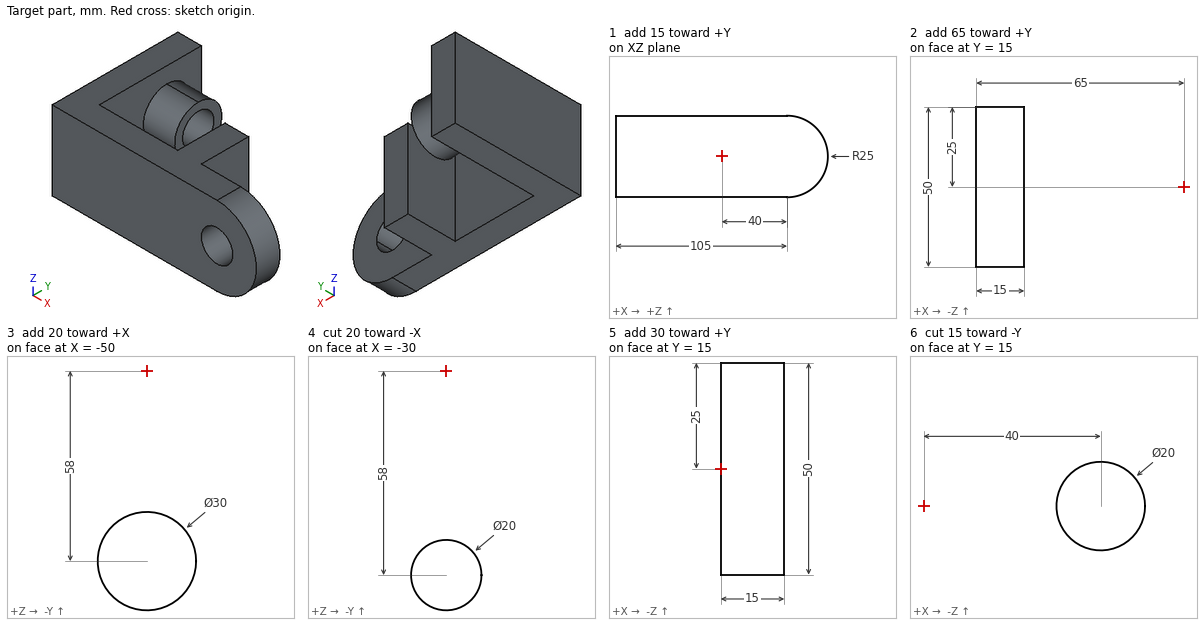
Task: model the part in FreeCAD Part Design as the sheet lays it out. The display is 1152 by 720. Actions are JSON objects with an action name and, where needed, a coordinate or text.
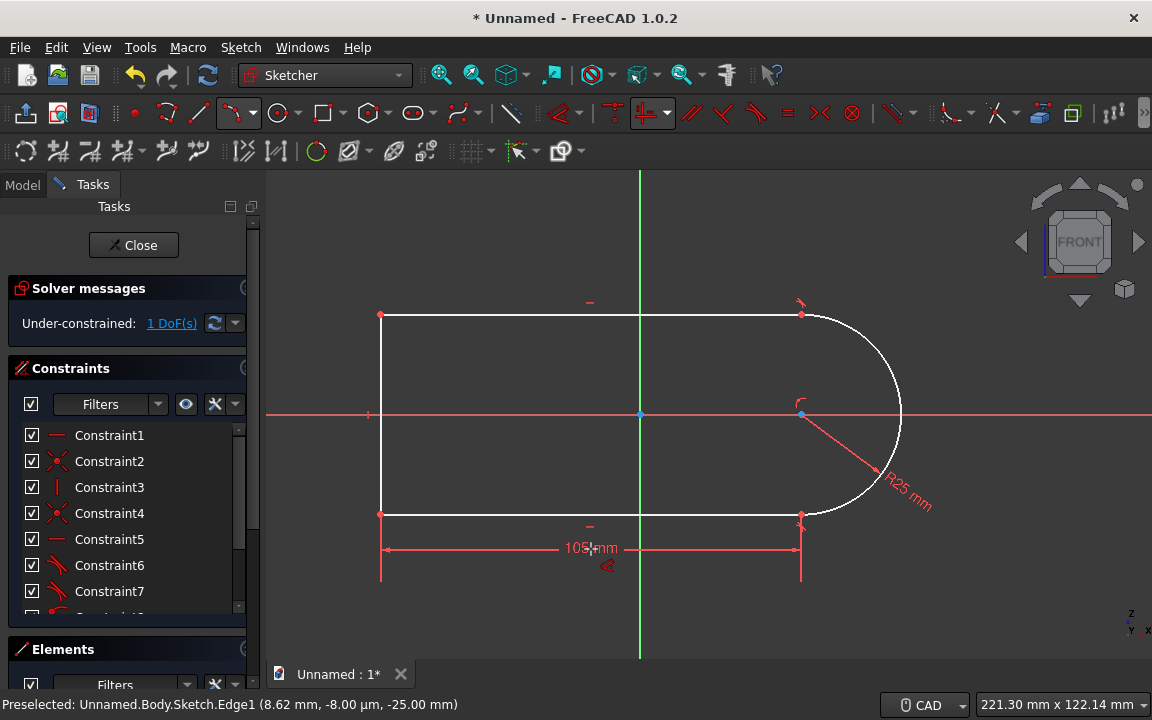
{"action": "left_click", "coordinate": [801, 515]}
{"action": "left_click", "coordinate": [721, 549]}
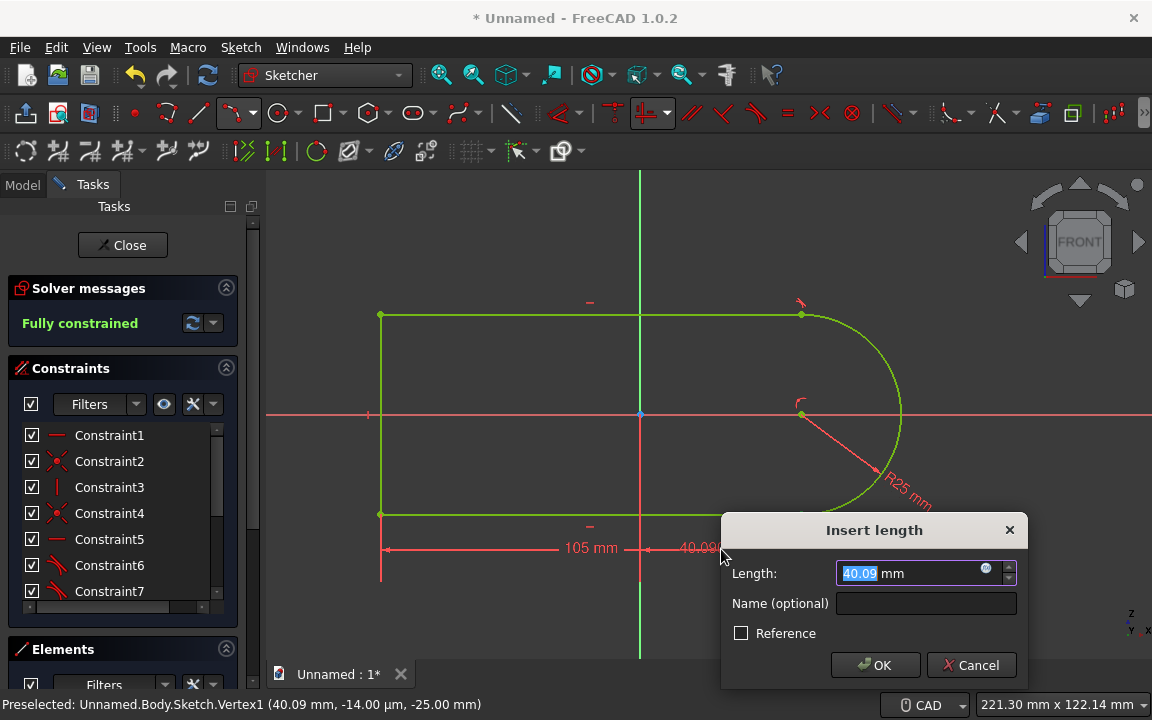
{"action": "type", "text": "40"}
{"action": "key", "text": "Return"}
{"action": "key", "text": "Escape"}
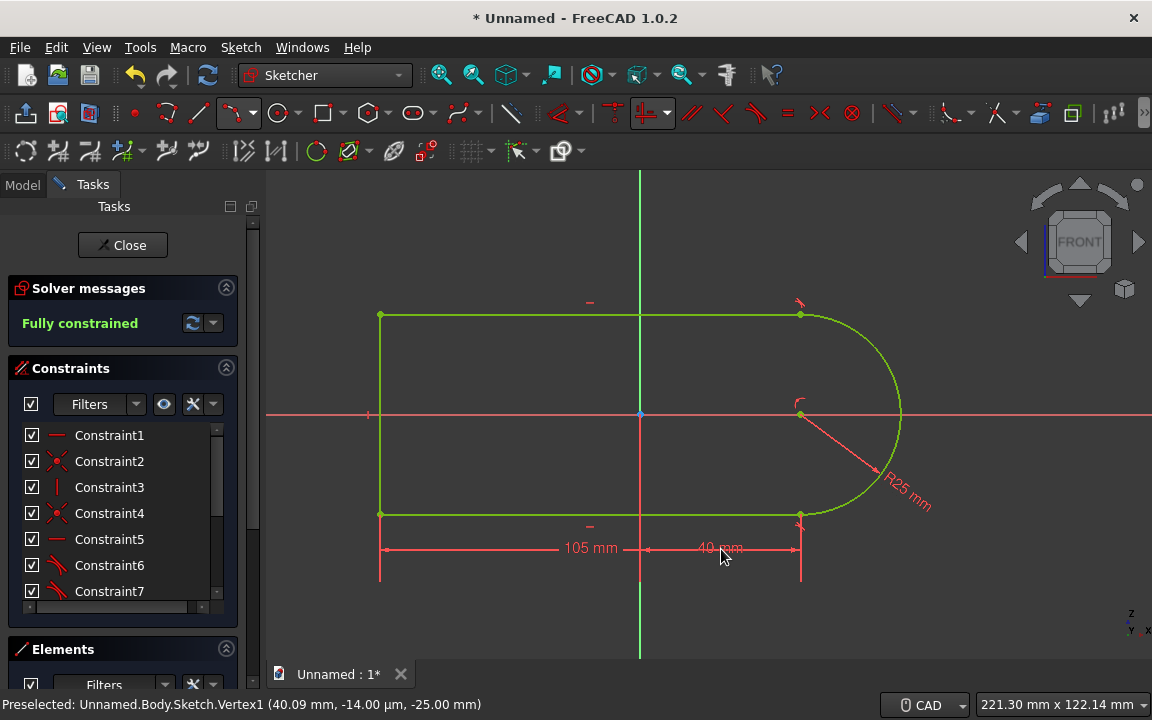
{"action": "left_click", "coordinate": [123, 245]}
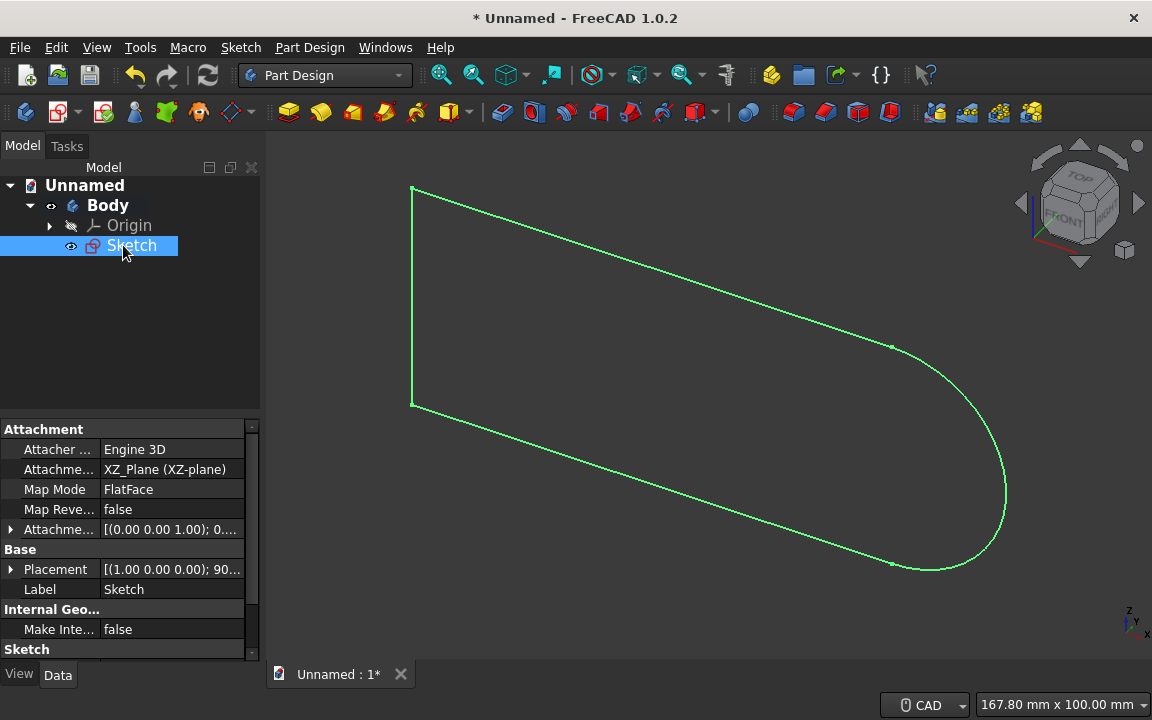
{"action": "left_click", "coordinate": [290, 112]}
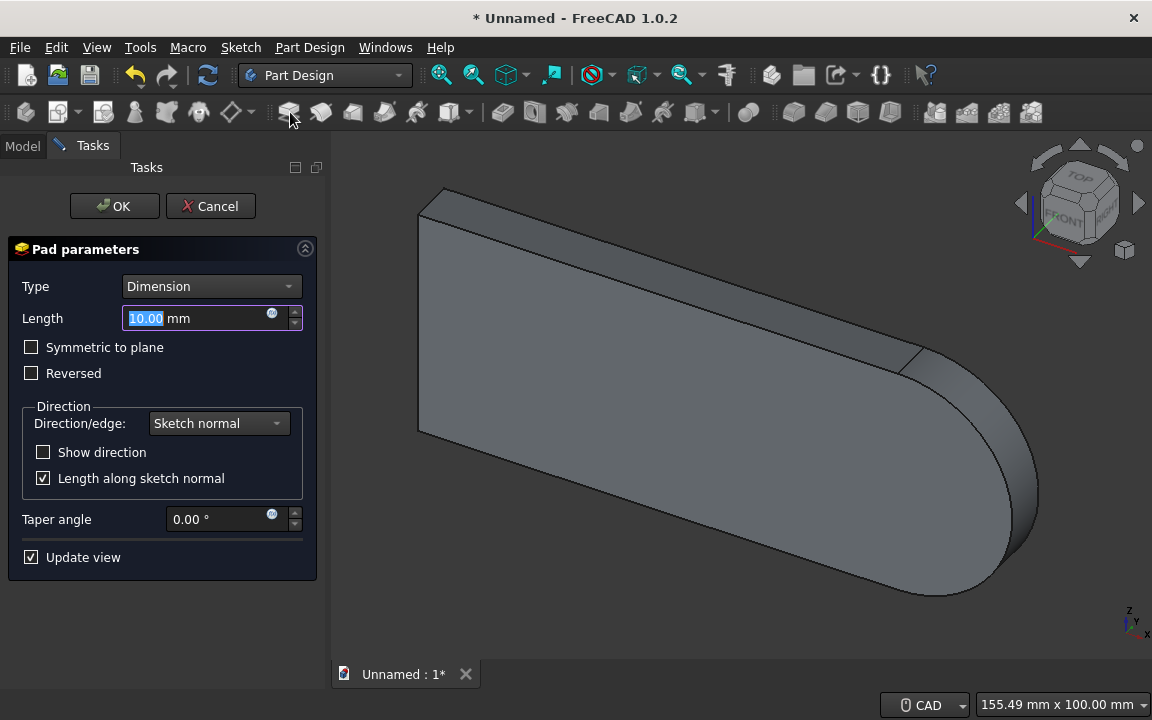
{"action": "type", "text": "15"}
{"action": "key", "text": "Tab"}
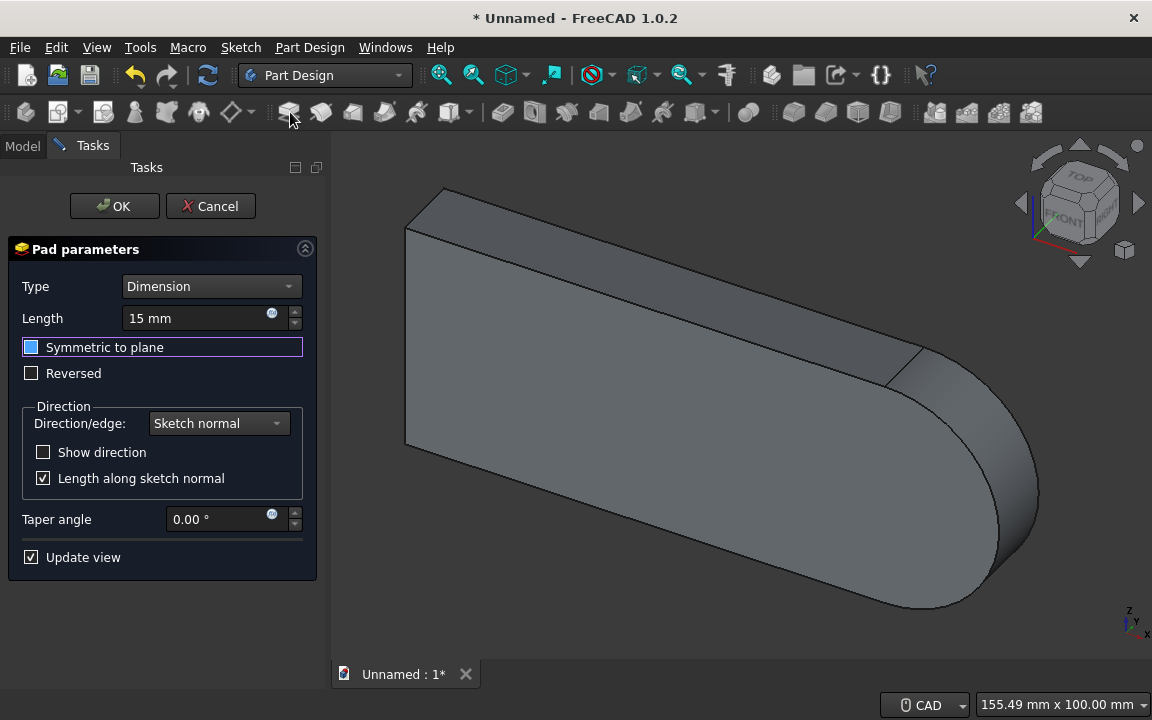
{"action": "left_click", "coordinate": [30, 373]}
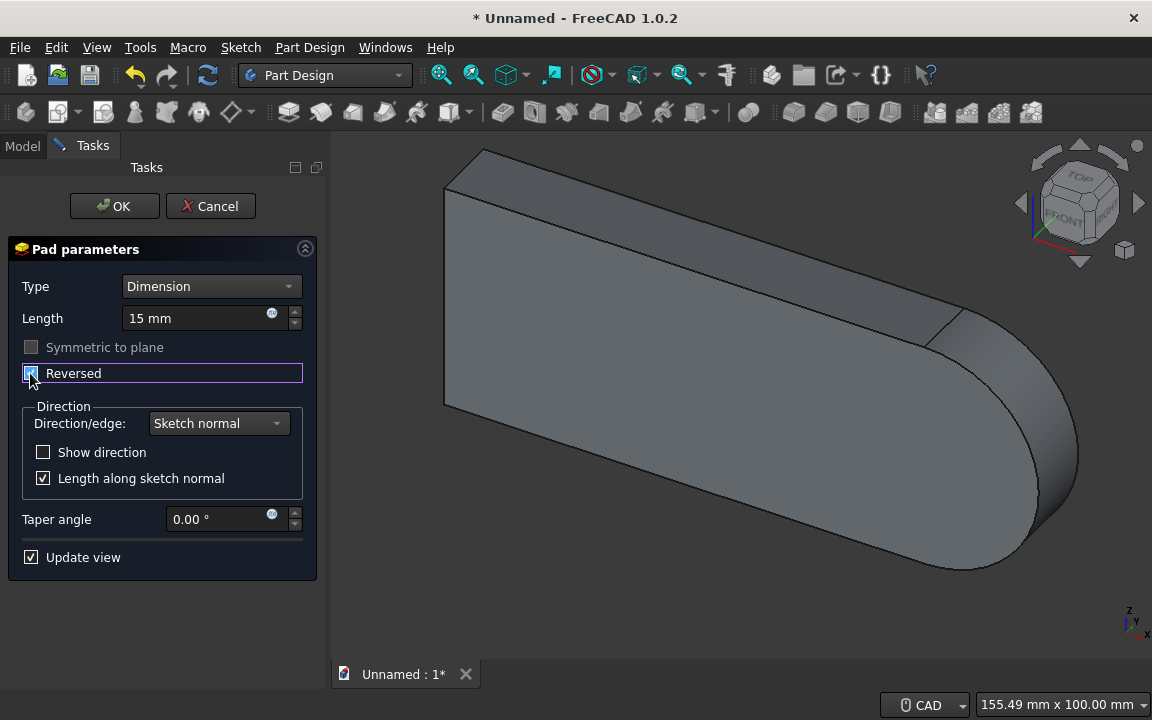
{"action": "left_click", "coordinate": [115, 206]}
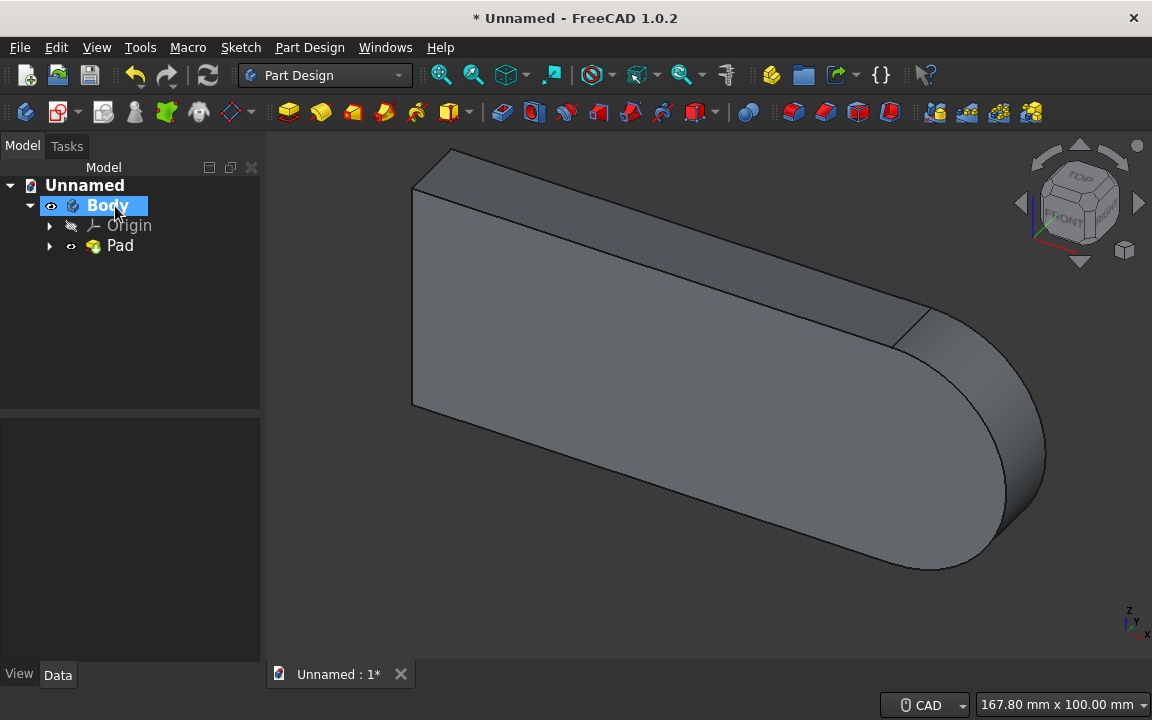
{"action": "key", "text": "4"}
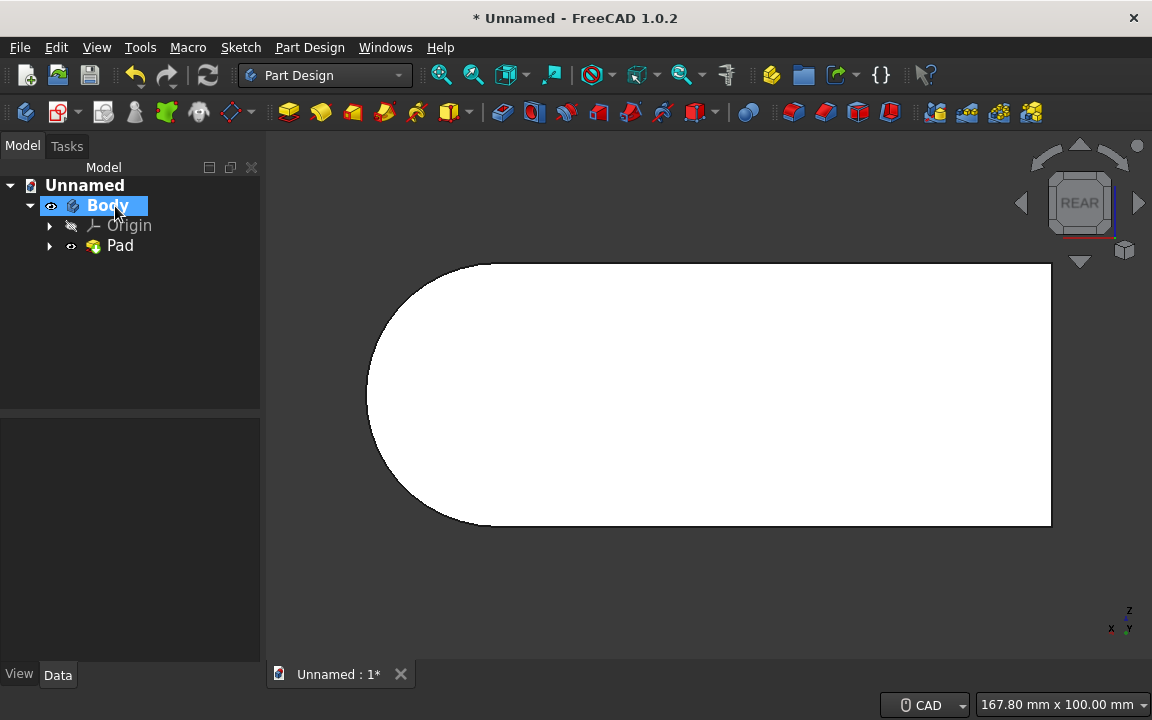
{"action": "left_click", "coordinate": [513, 394]}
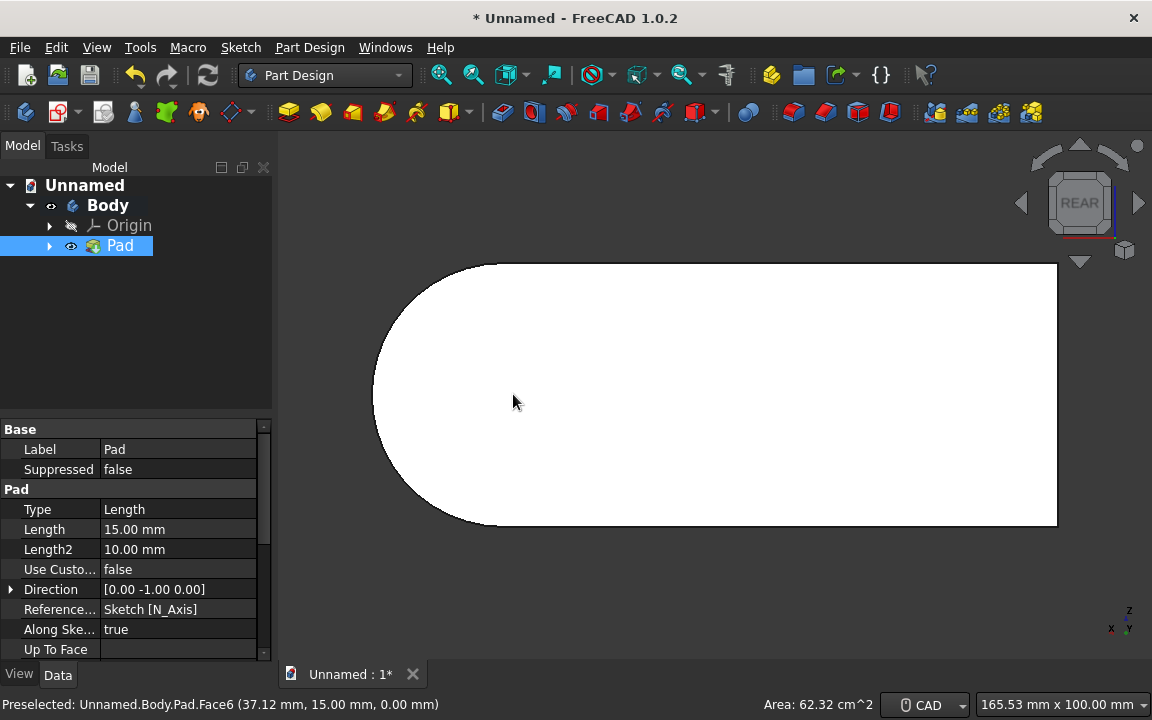
{"action": "left_click", "coordinate": [58, 112]}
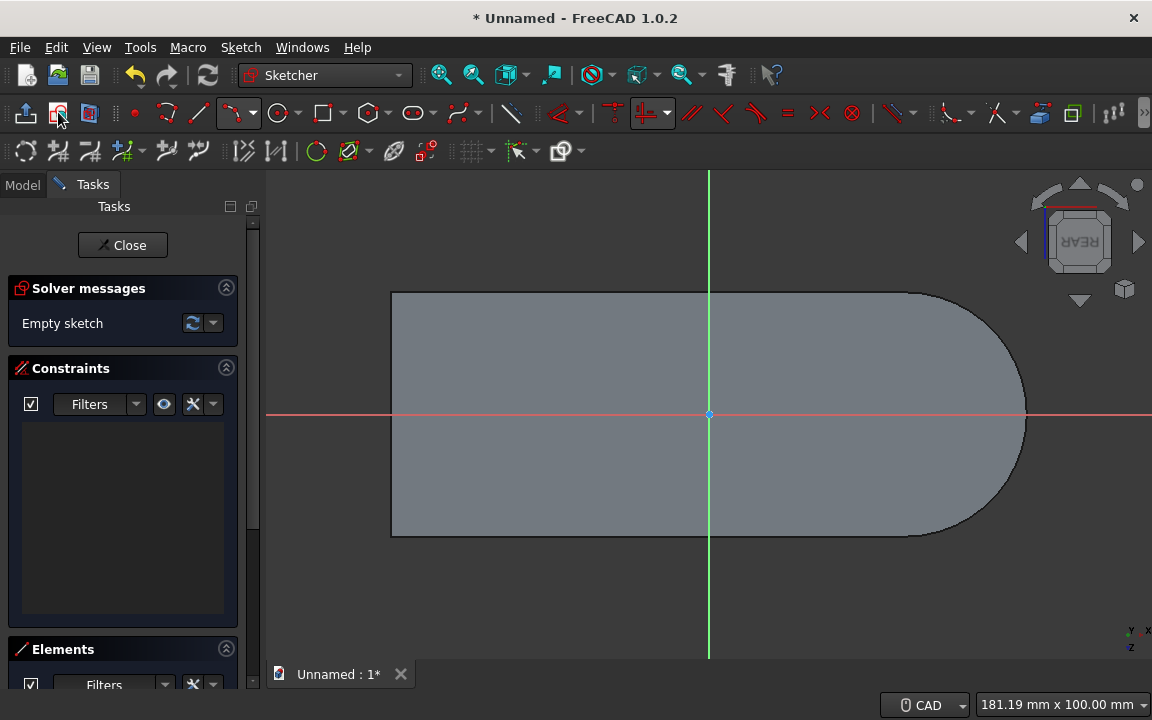
{"action": "left_click", "coordinate": [324, 114]}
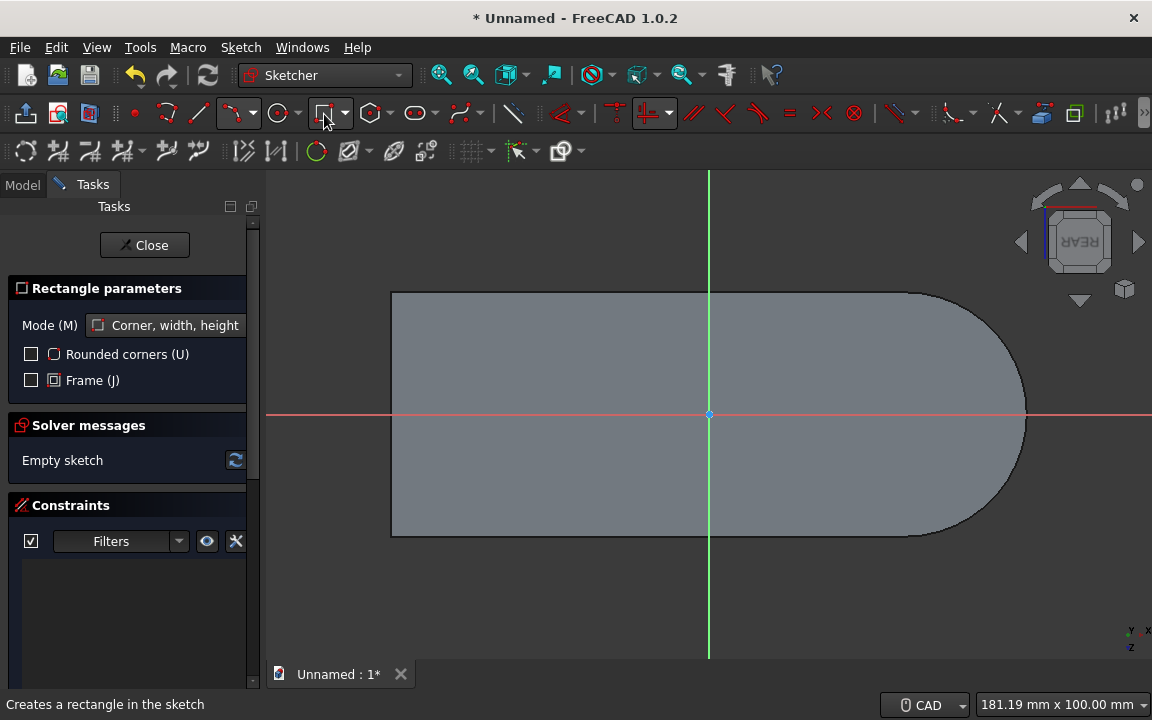
{"action": "left_click", "coordinate": [391, 292]}
{"action": "mouse_move", "coordinate": [464, 537]}